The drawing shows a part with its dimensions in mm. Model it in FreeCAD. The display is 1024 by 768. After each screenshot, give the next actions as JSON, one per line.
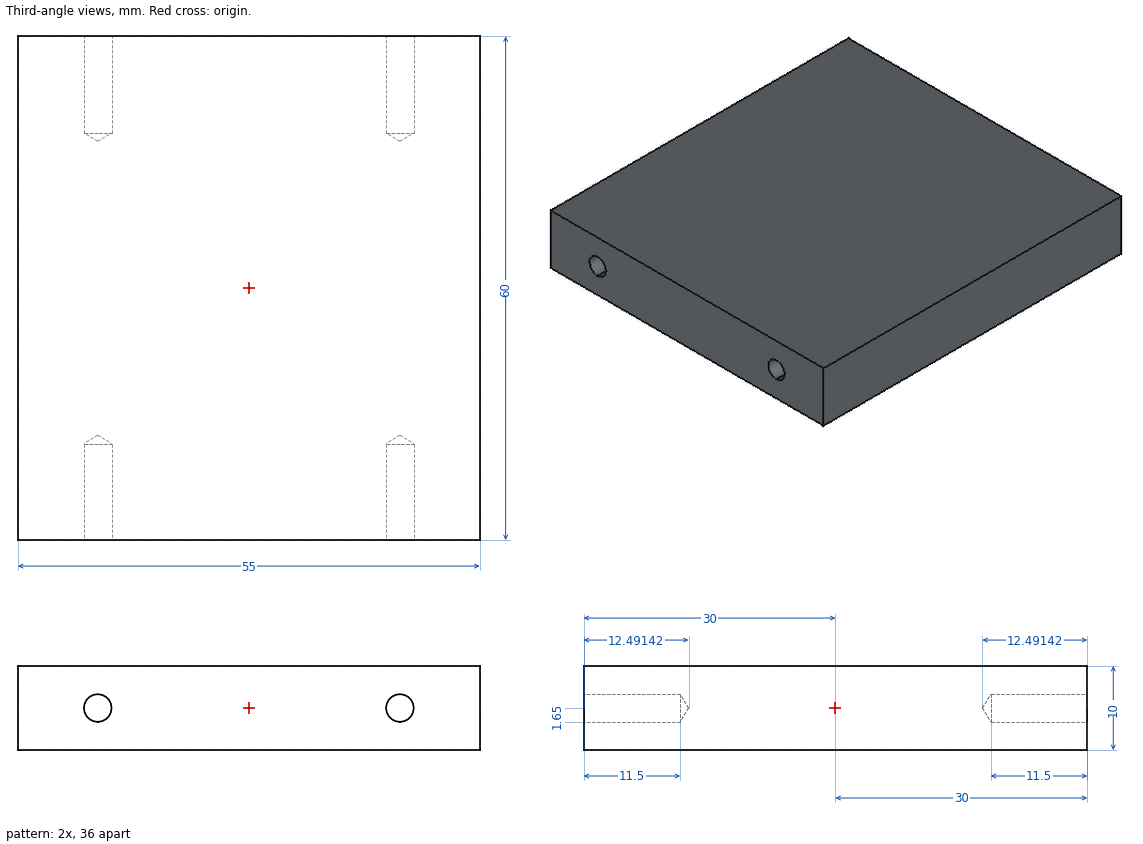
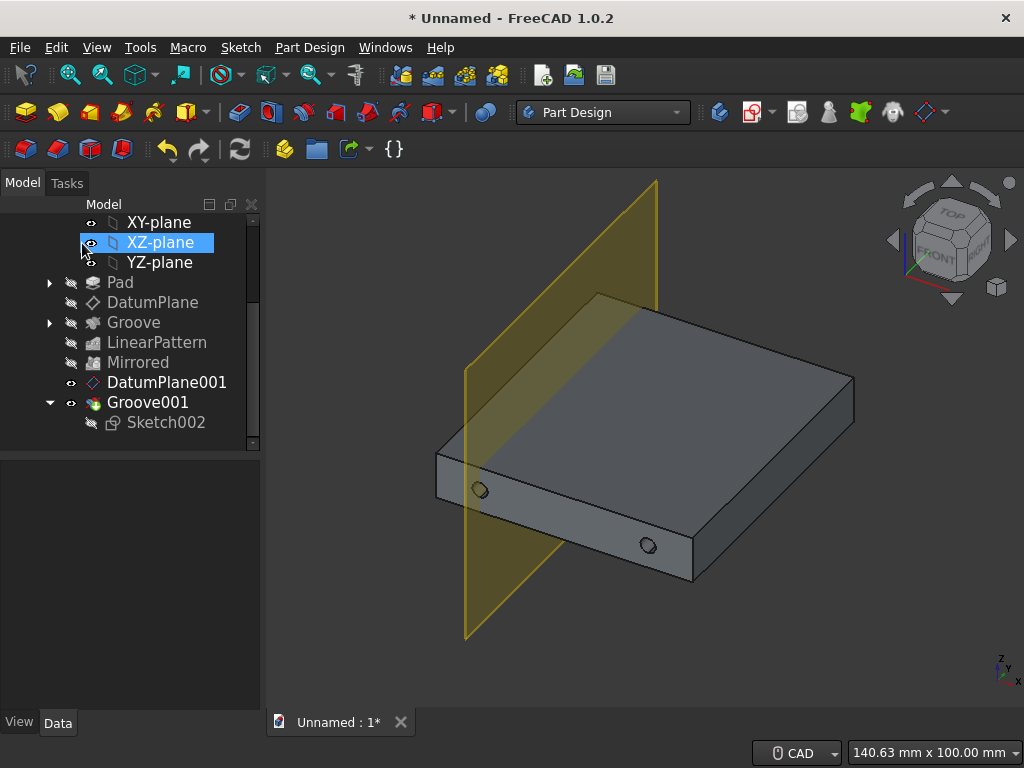
{"action": "left_click", "coordinate": [116, 383]}
{"action": "key", "text": "space"}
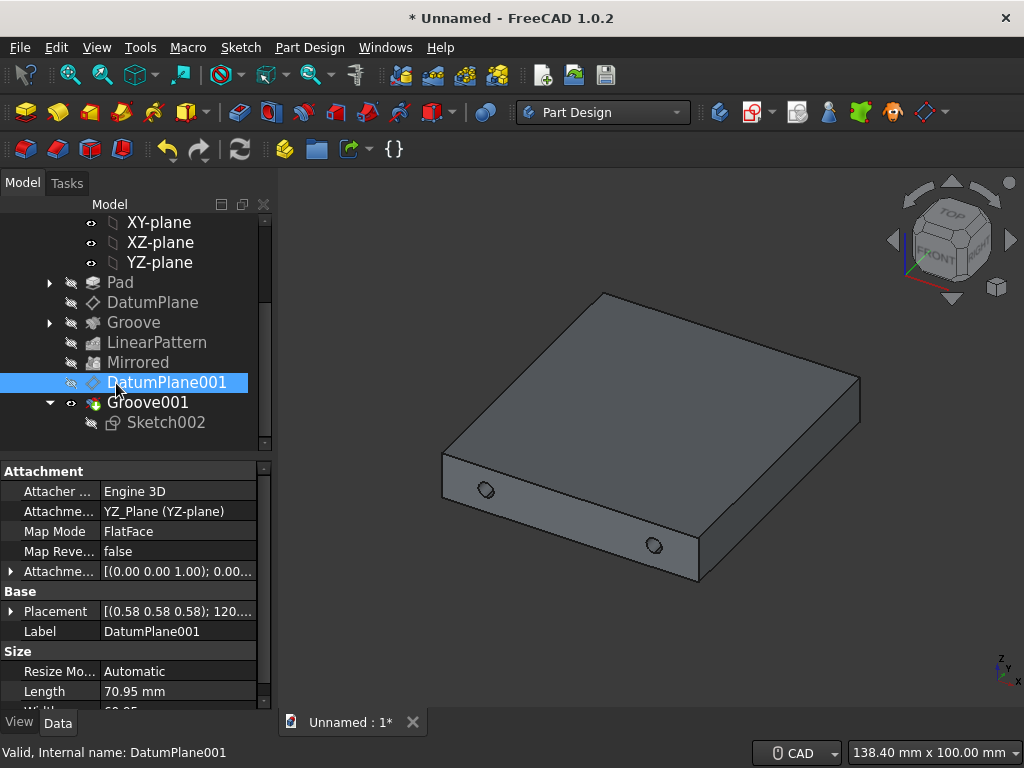
{"action": "key", "text": "0"}